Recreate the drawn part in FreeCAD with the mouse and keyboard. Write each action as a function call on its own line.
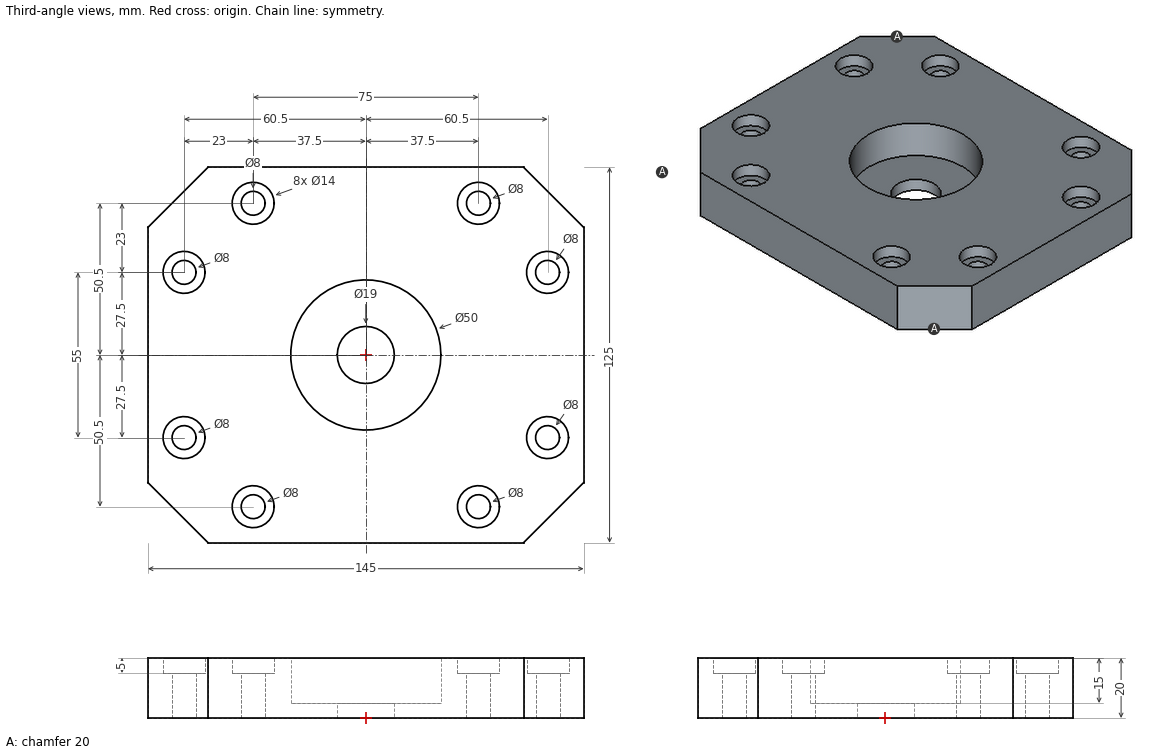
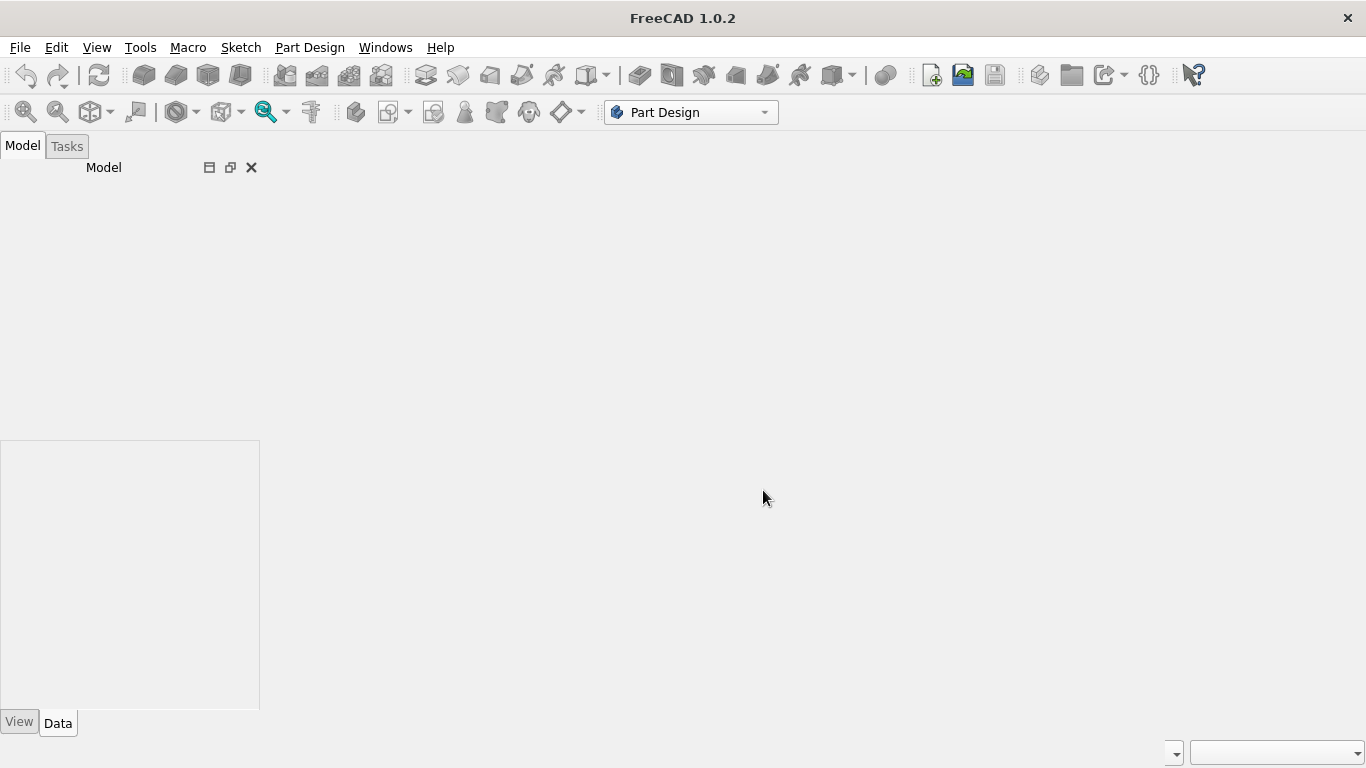
click(932, 76)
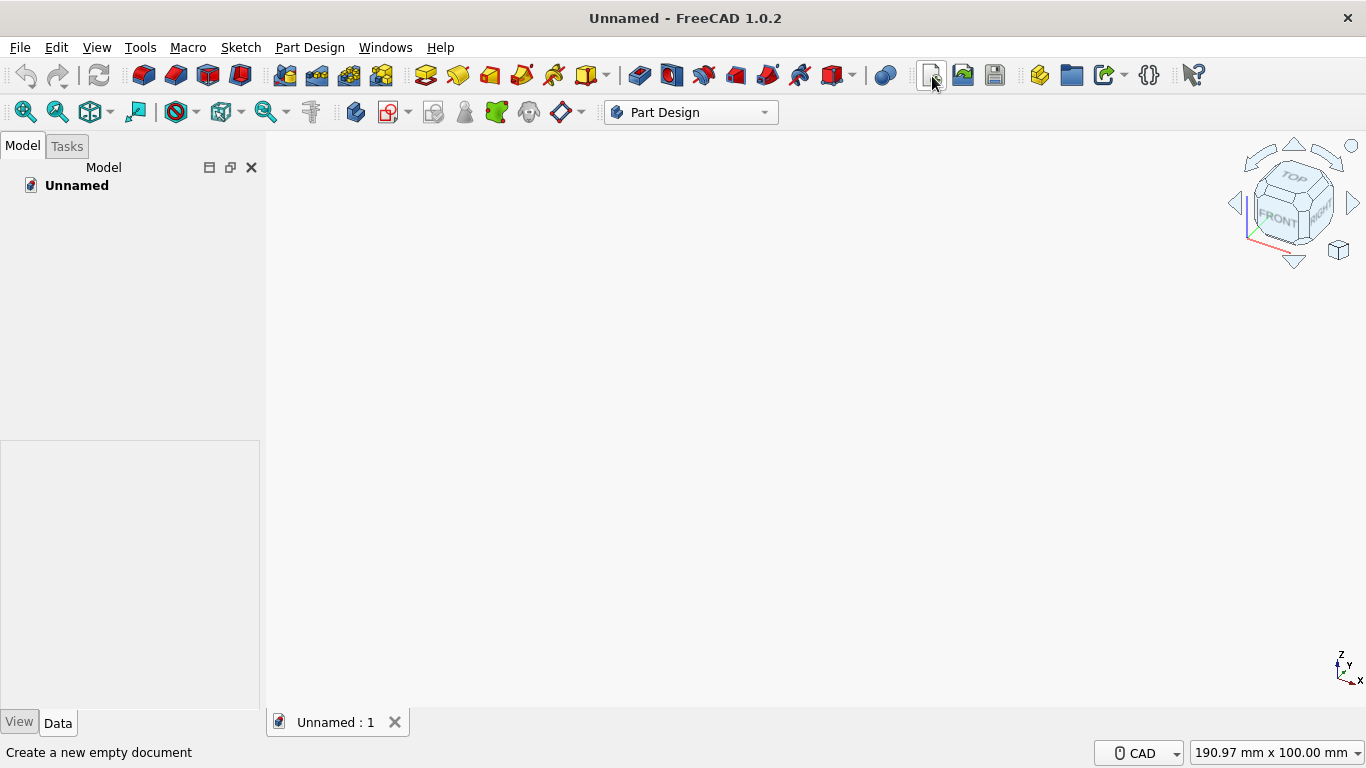
click(388, 112)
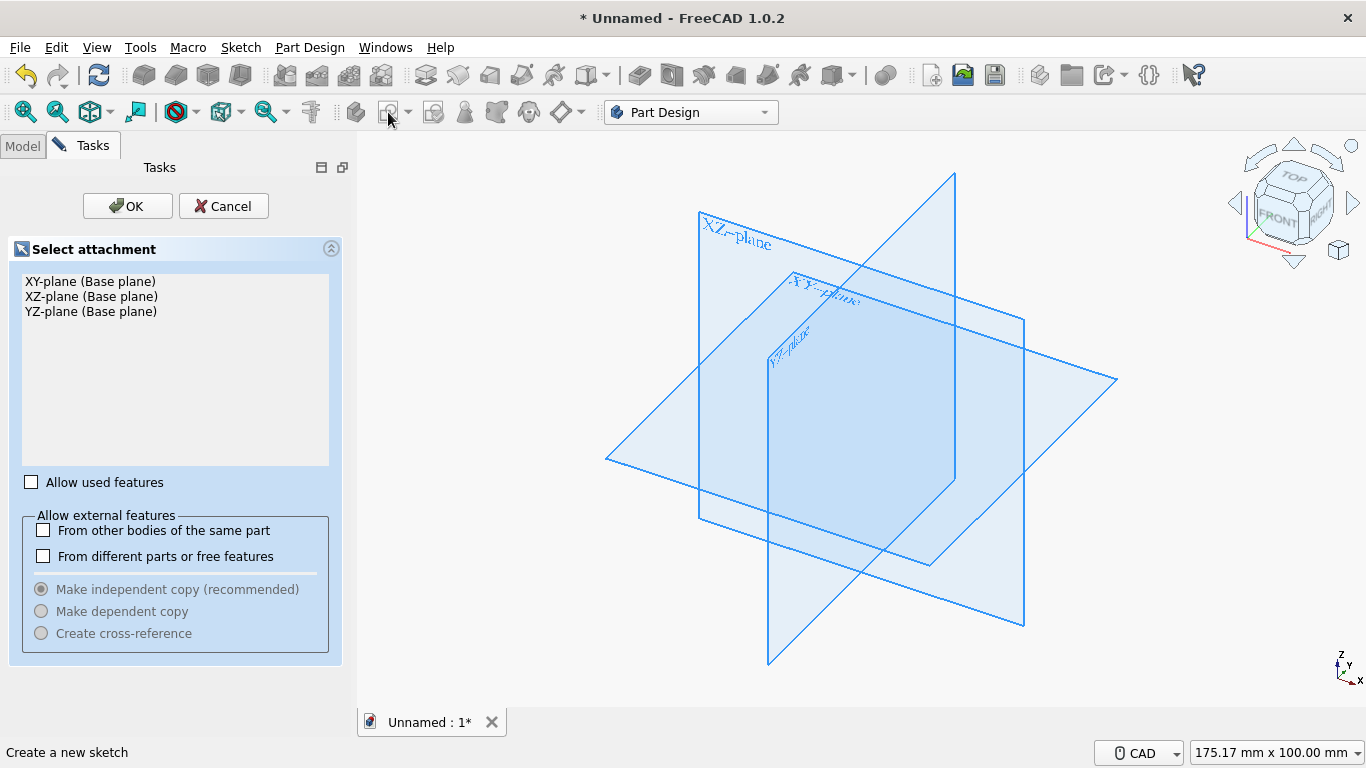
click(82, 282)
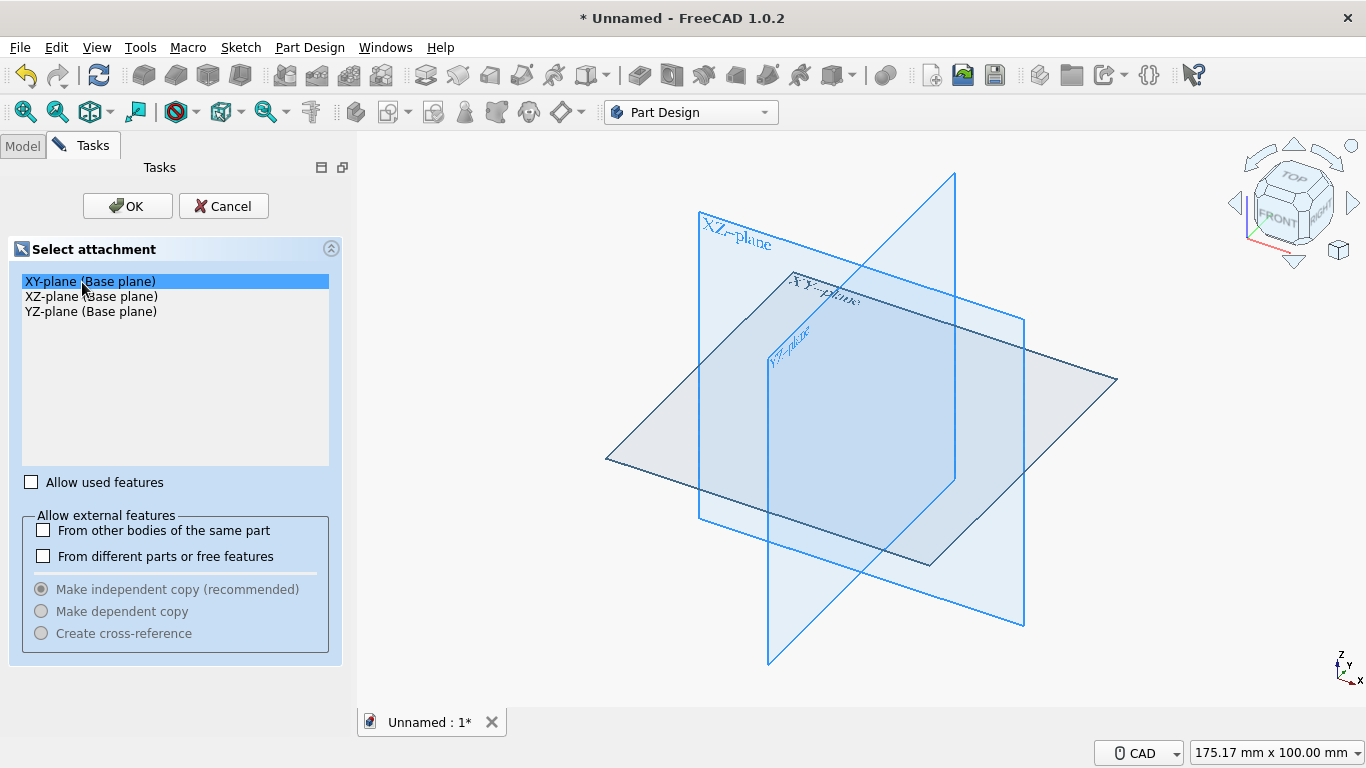
click(128, 206)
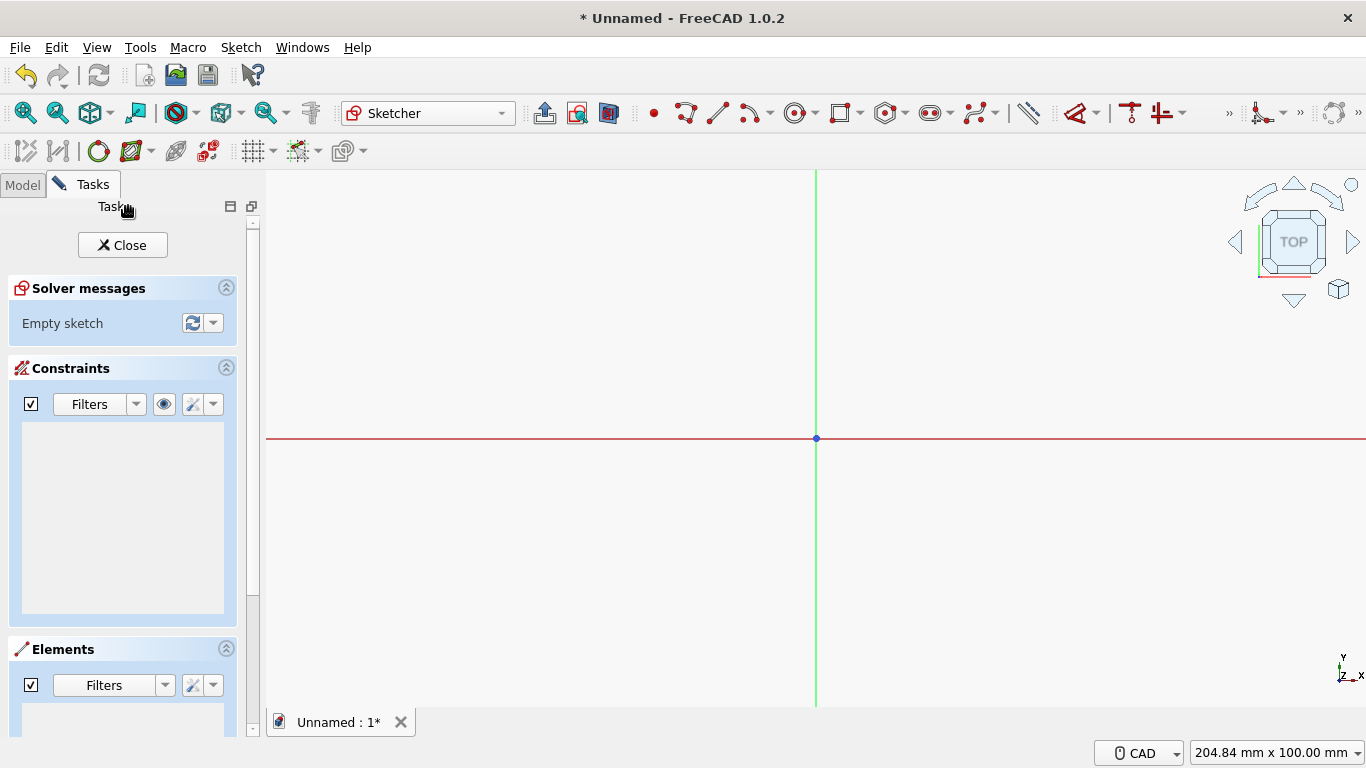
scroll(664, 438, down, 3)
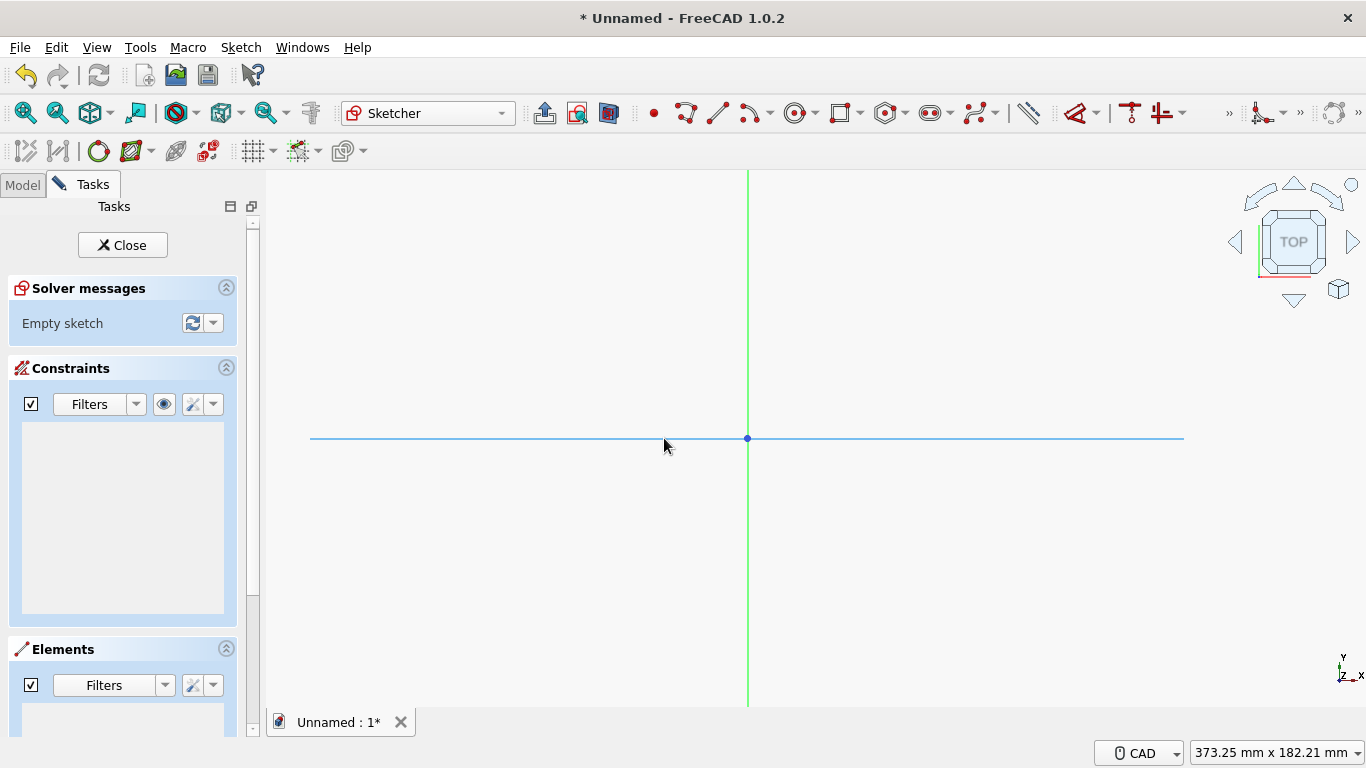
key(g)
key(v)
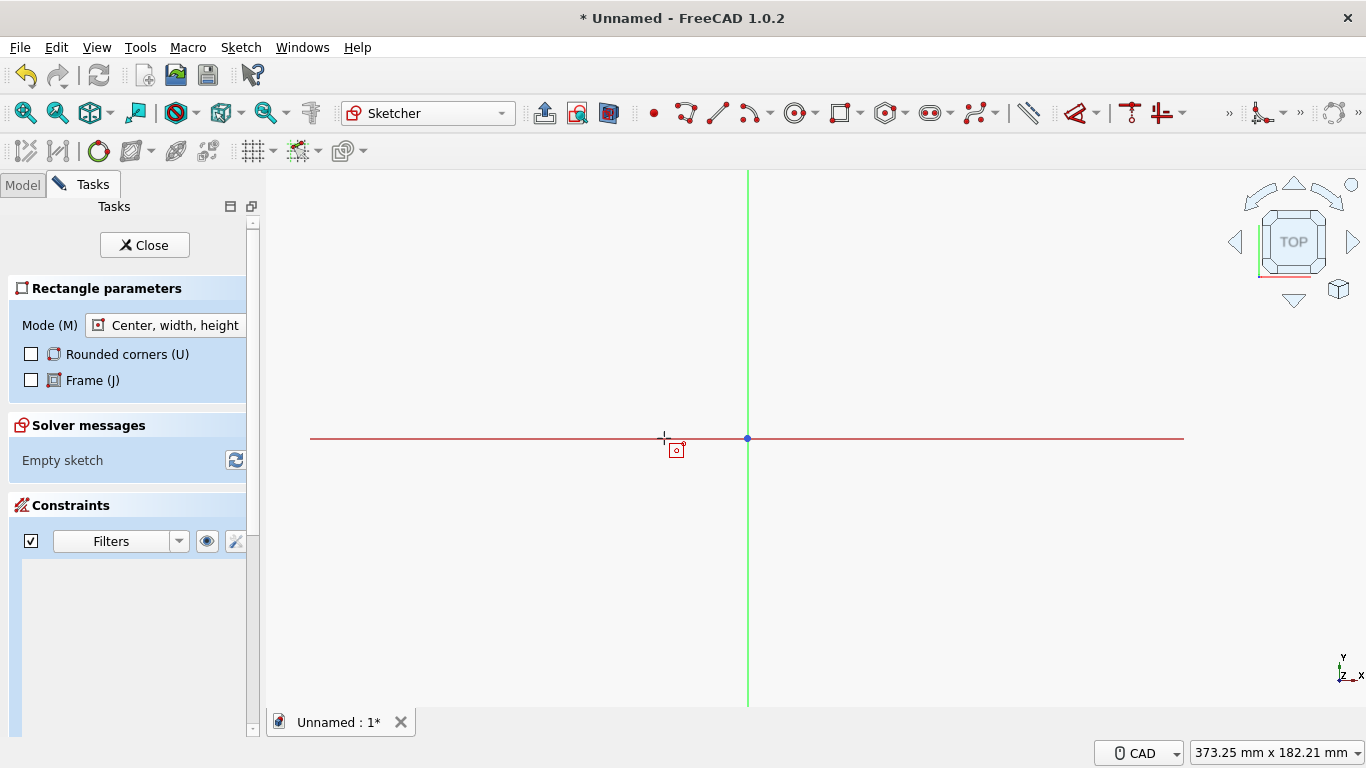
click(748, 438)
click(961, 254)
key(Escape)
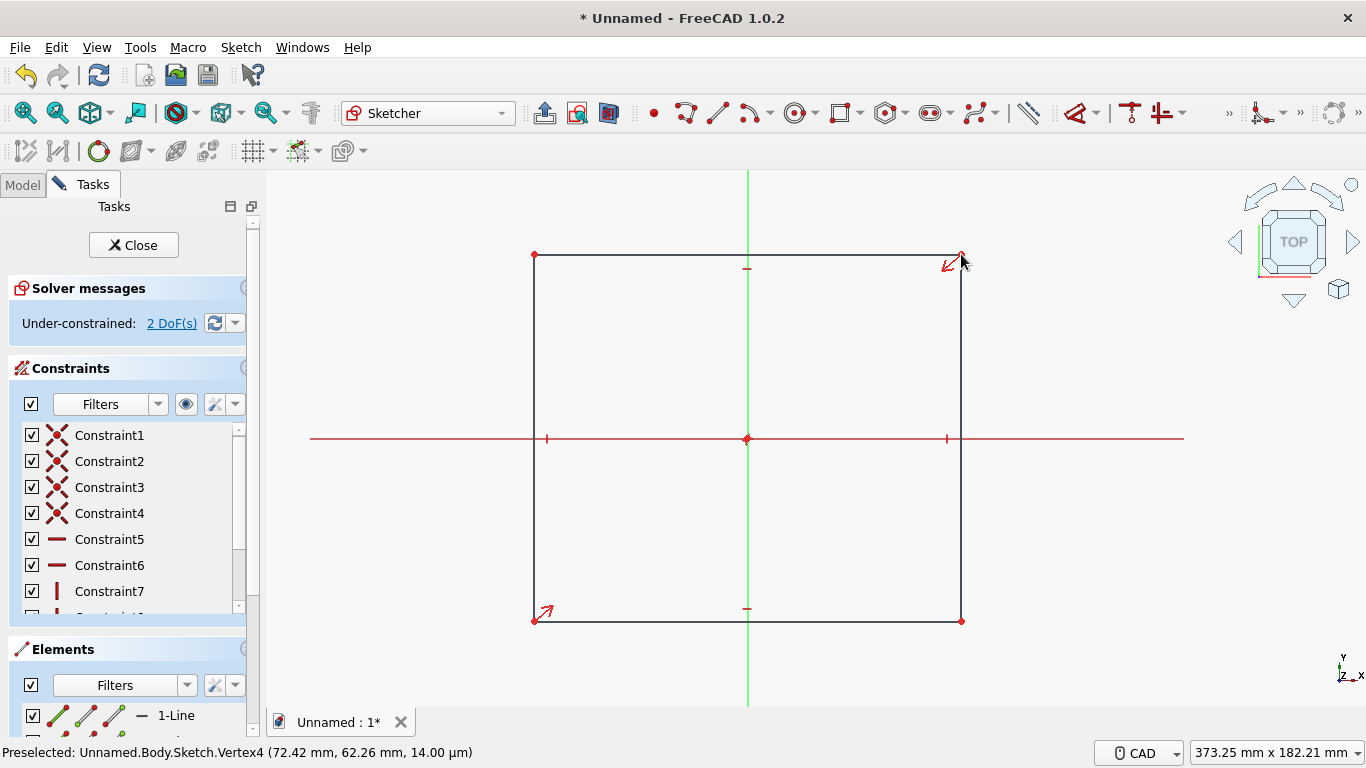
click(1076, 114)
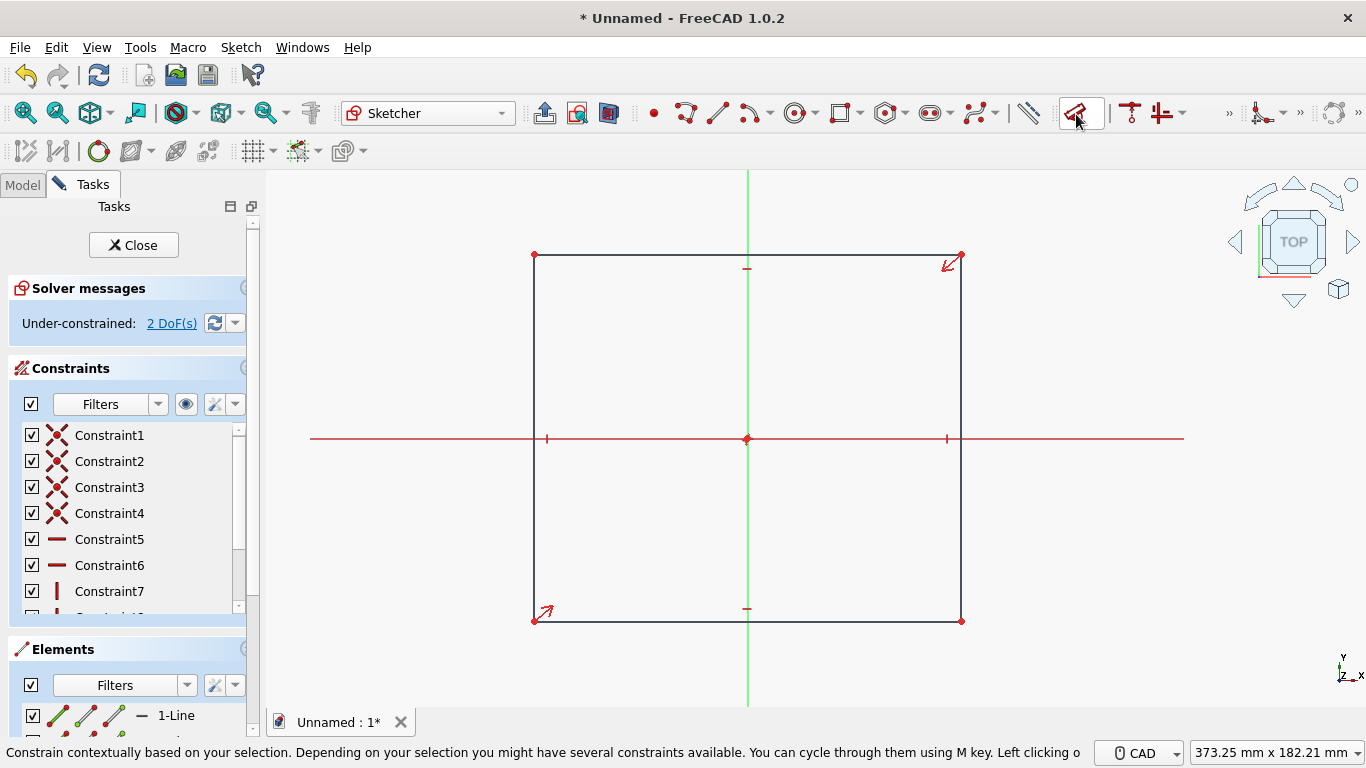
click(662, 622)
click(649, 656)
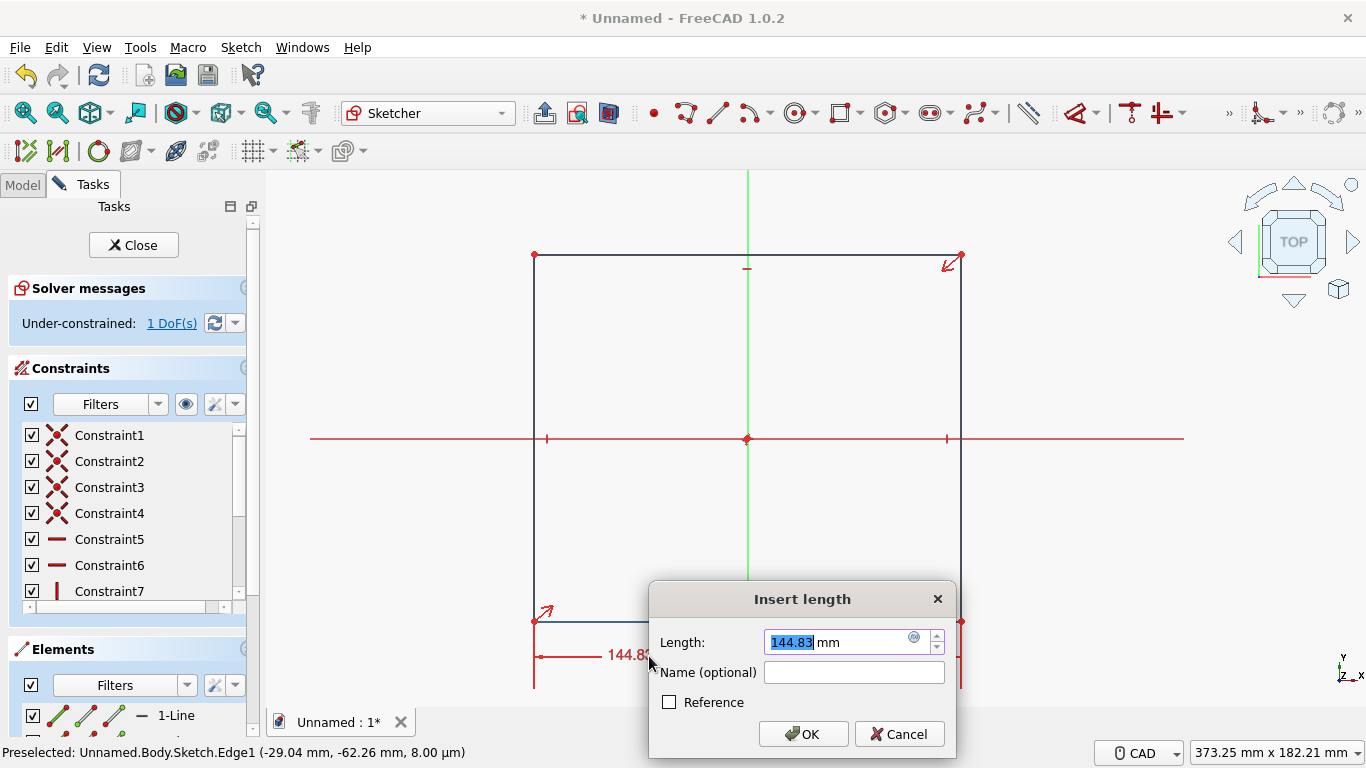
text(145)
key(Return)